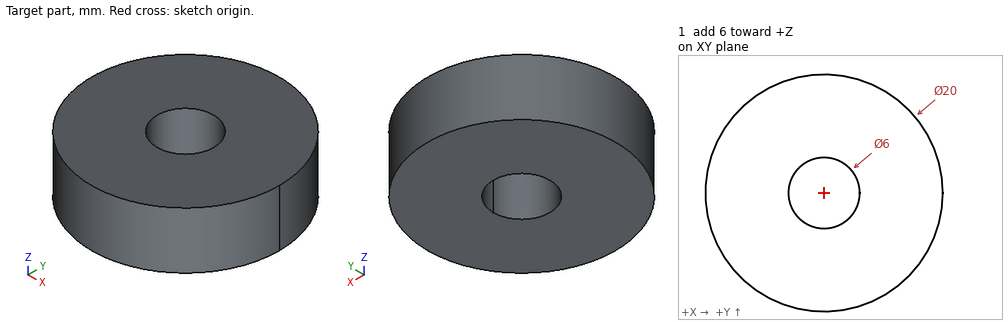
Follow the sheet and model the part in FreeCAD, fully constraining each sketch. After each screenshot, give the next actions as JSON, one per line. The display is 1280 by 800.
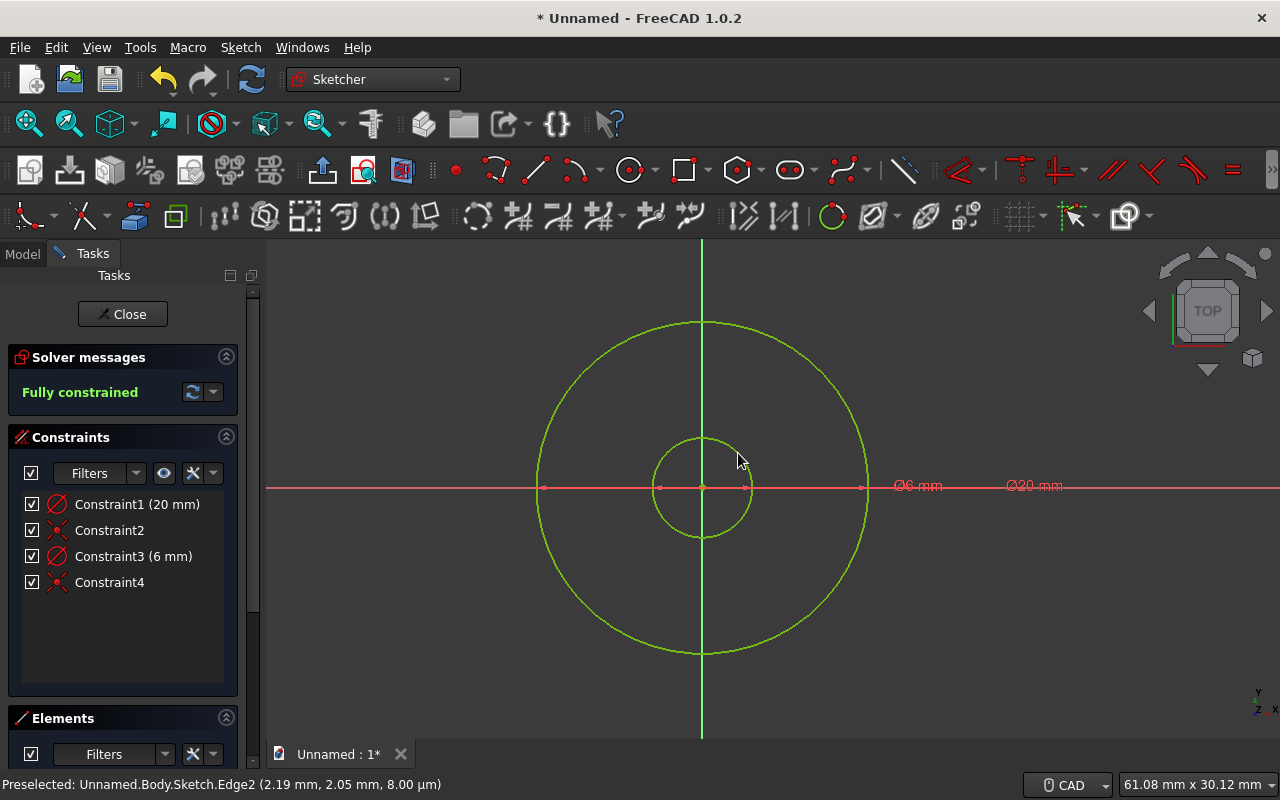
{"action": "left_click", "coordinate": [123, 314]}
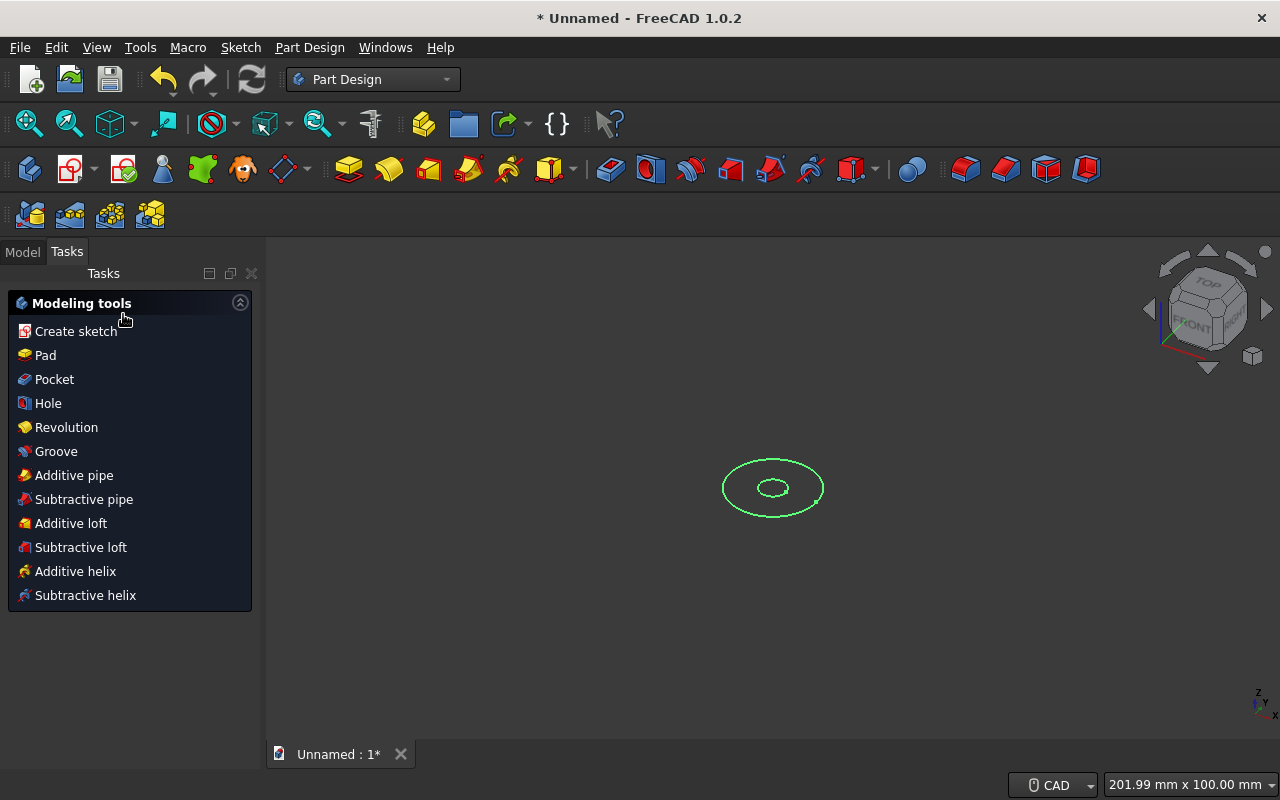
{"action": "left_click", "coordinate": [350, 170]}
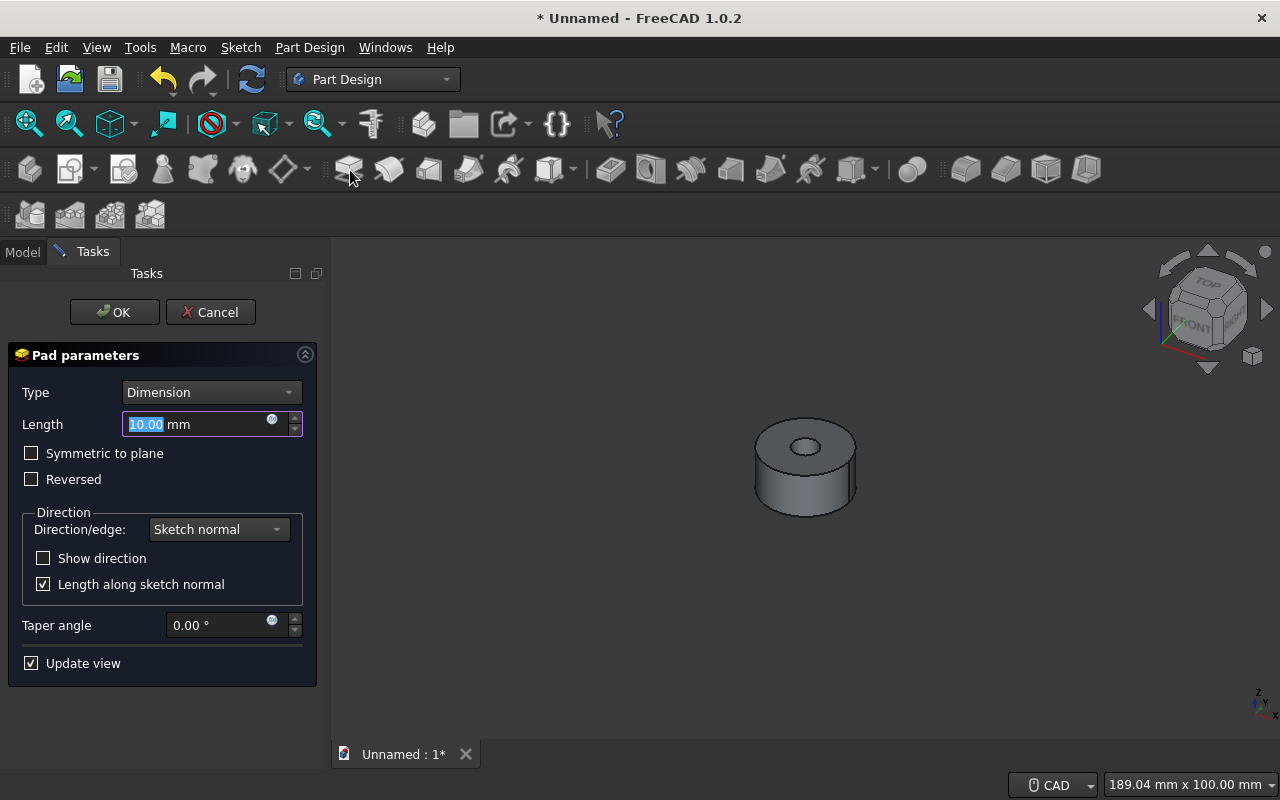
{"action": "type", "text": "6"}
{"action": "key", "text": "Tab"}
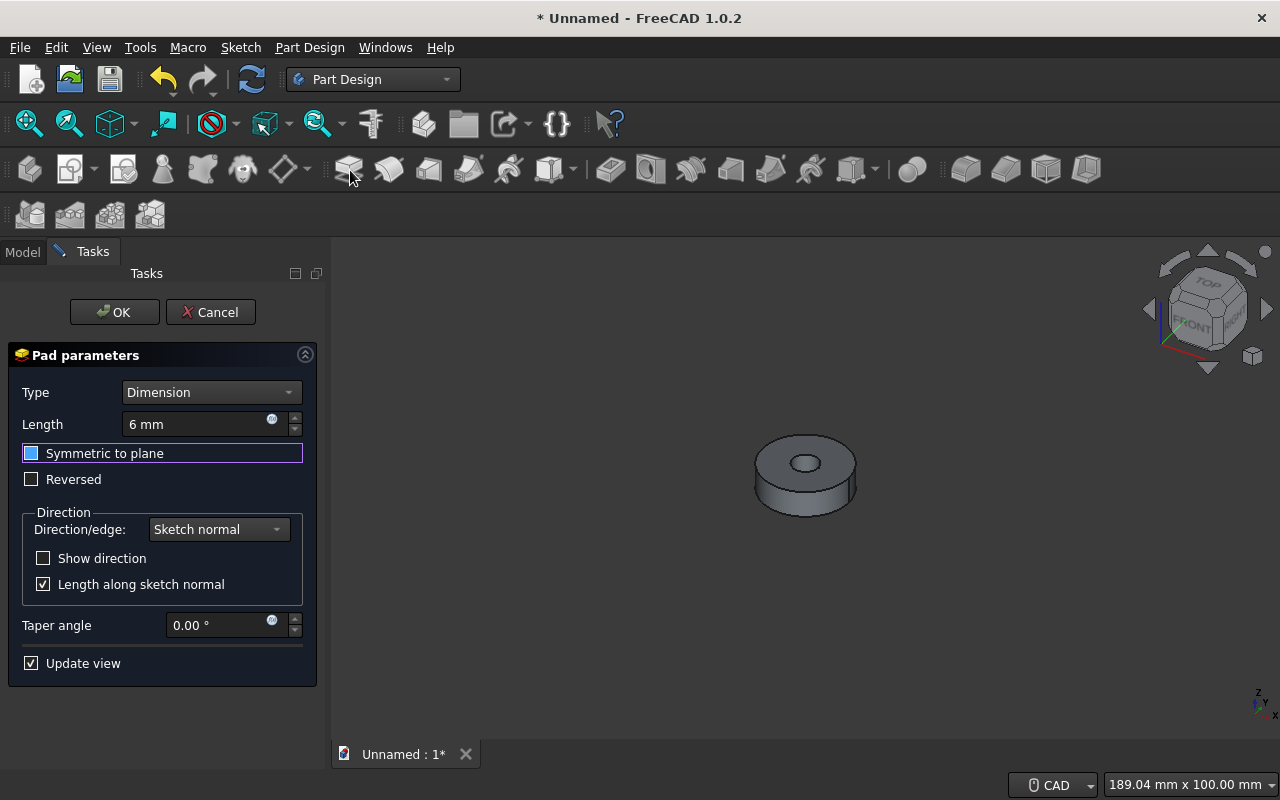
{"action": "left_click", "coordinate": [115, 312]}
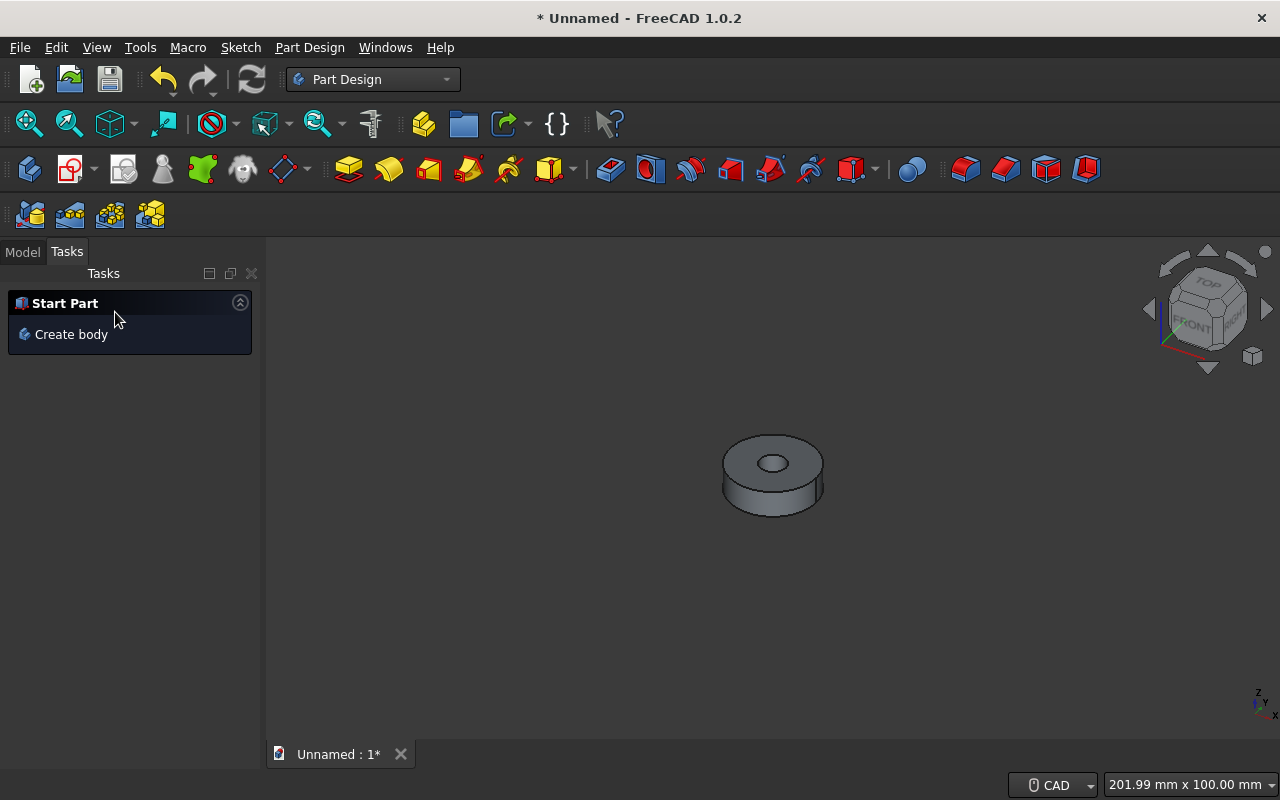
{"action": "key", "text": "0"}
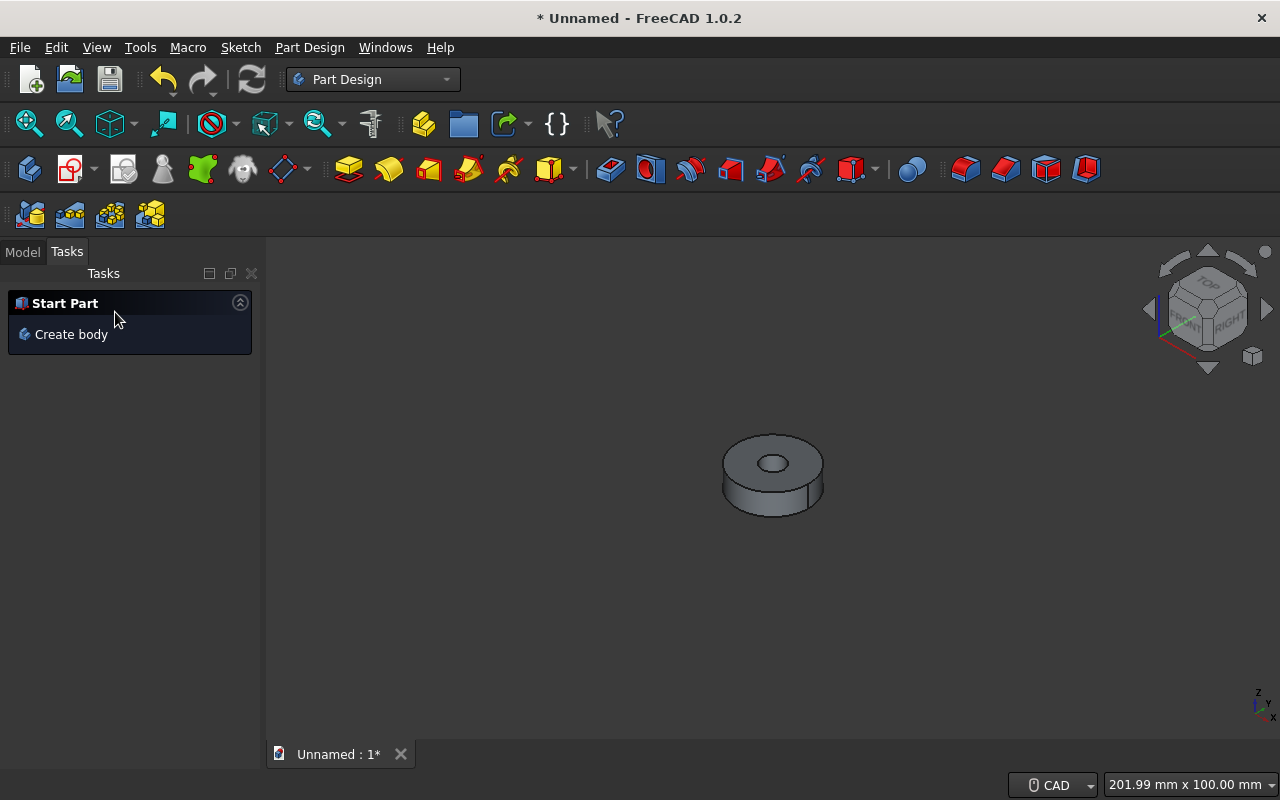
{"action": "left_click", "coordinate": [30, 124]}